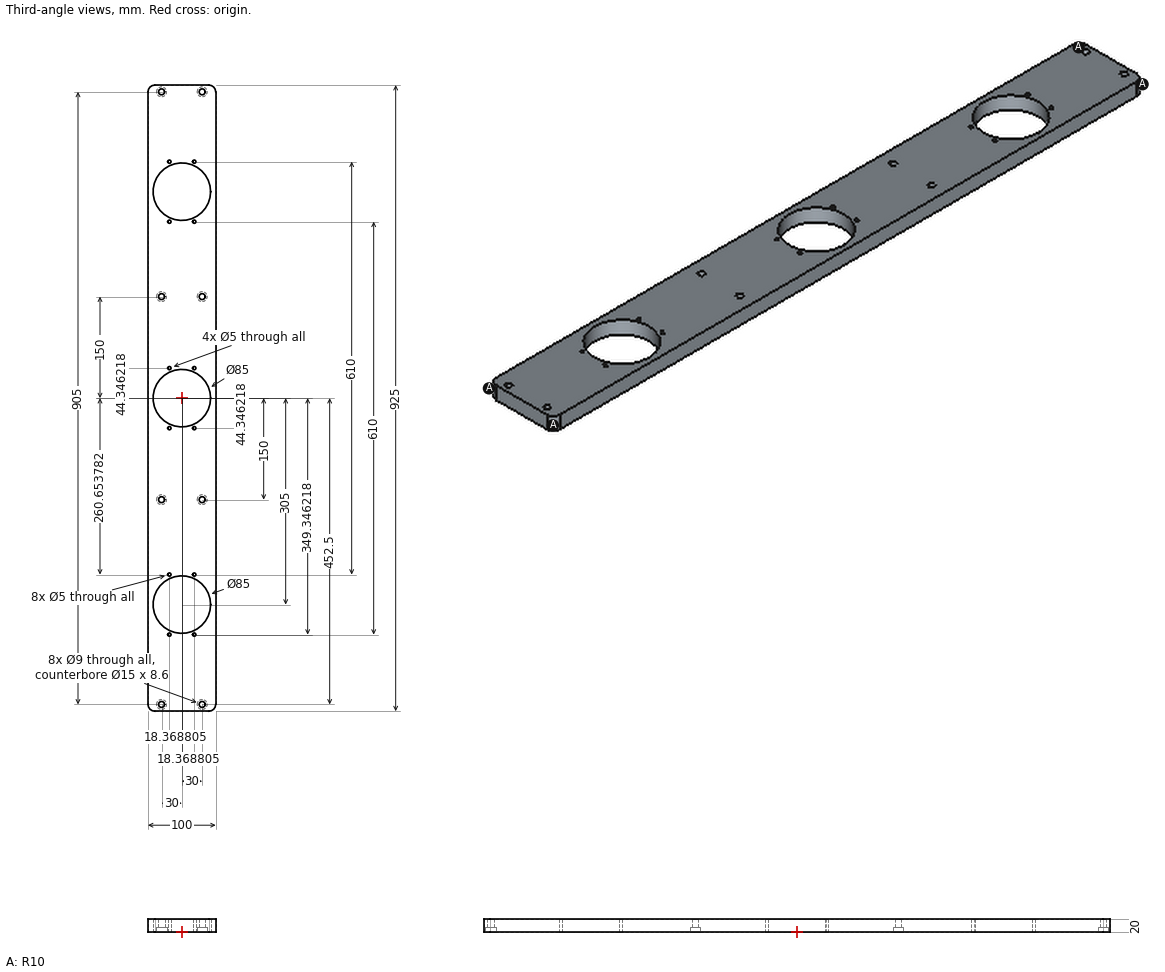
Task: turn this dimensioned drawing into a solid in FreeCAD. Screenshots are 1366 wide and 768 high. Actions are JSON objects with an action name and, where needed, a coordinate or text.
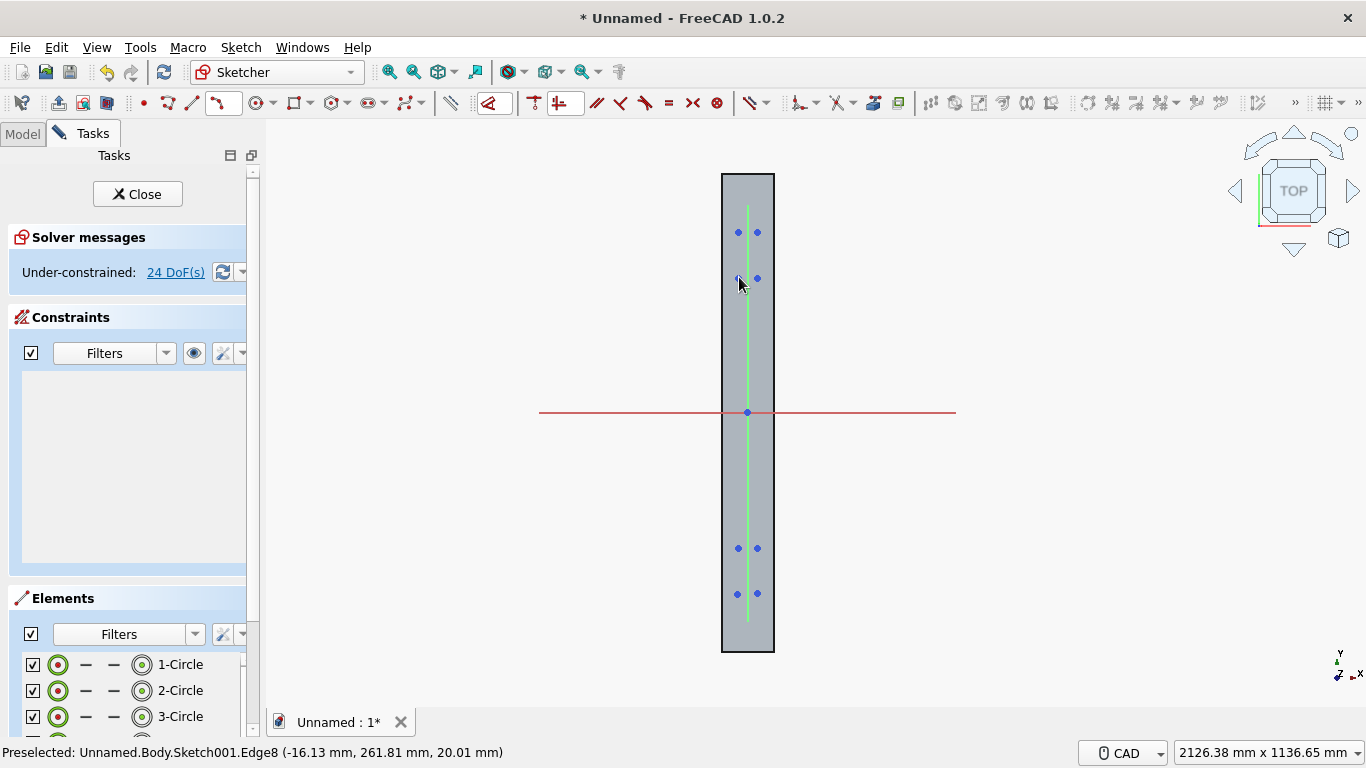
{"action": "scroll", "coordinate": [739, 547], "scroll_direction": "up", "scroll_amount": 11}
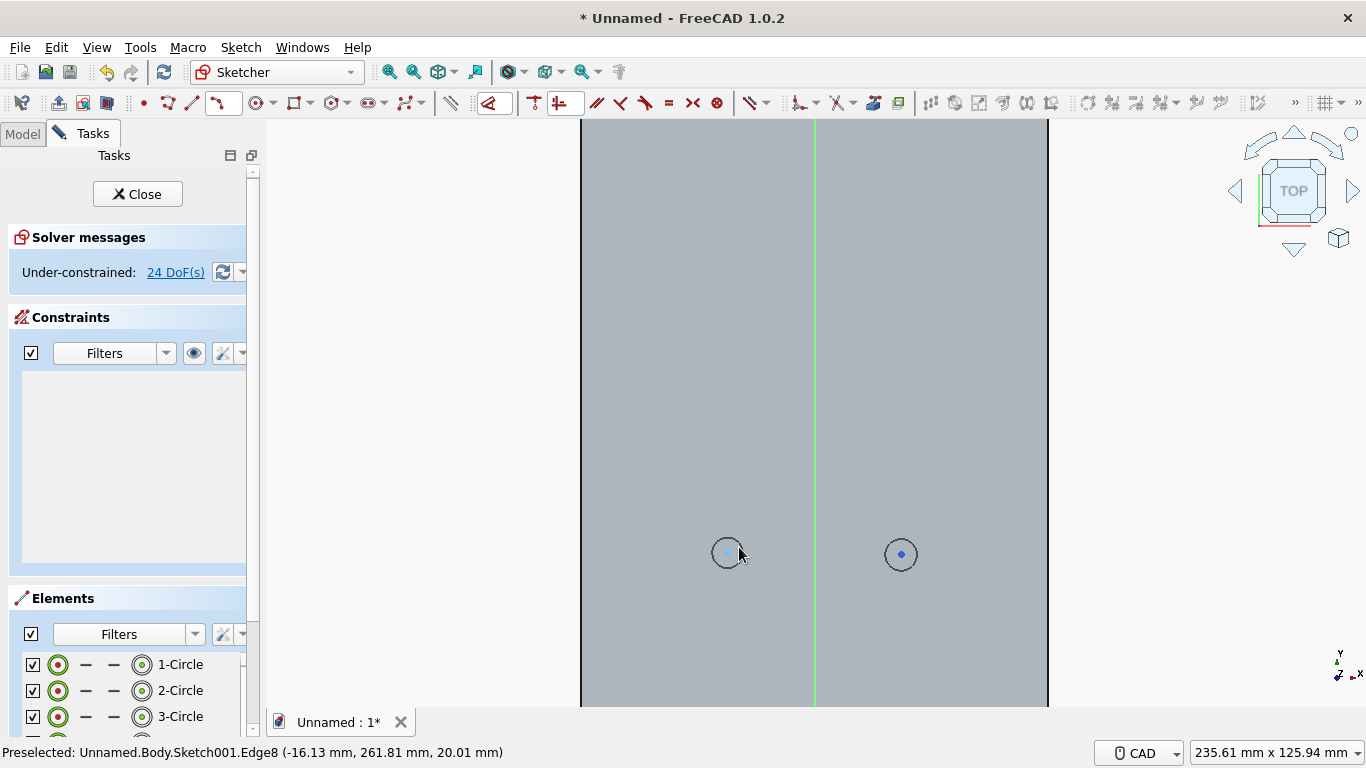
{"action": "left_click", "coordinate": [738, 542]}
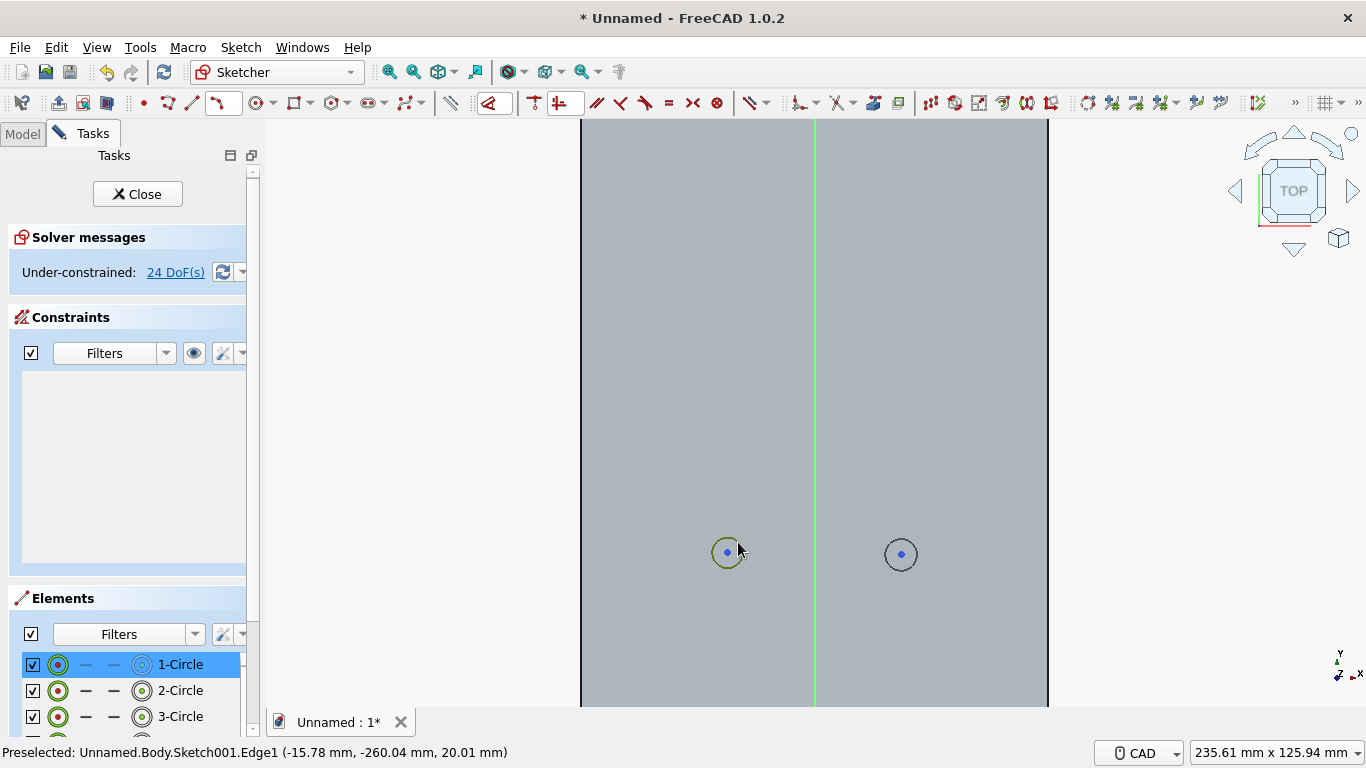
{"action": "left_click", "coordinate": [912, 544]}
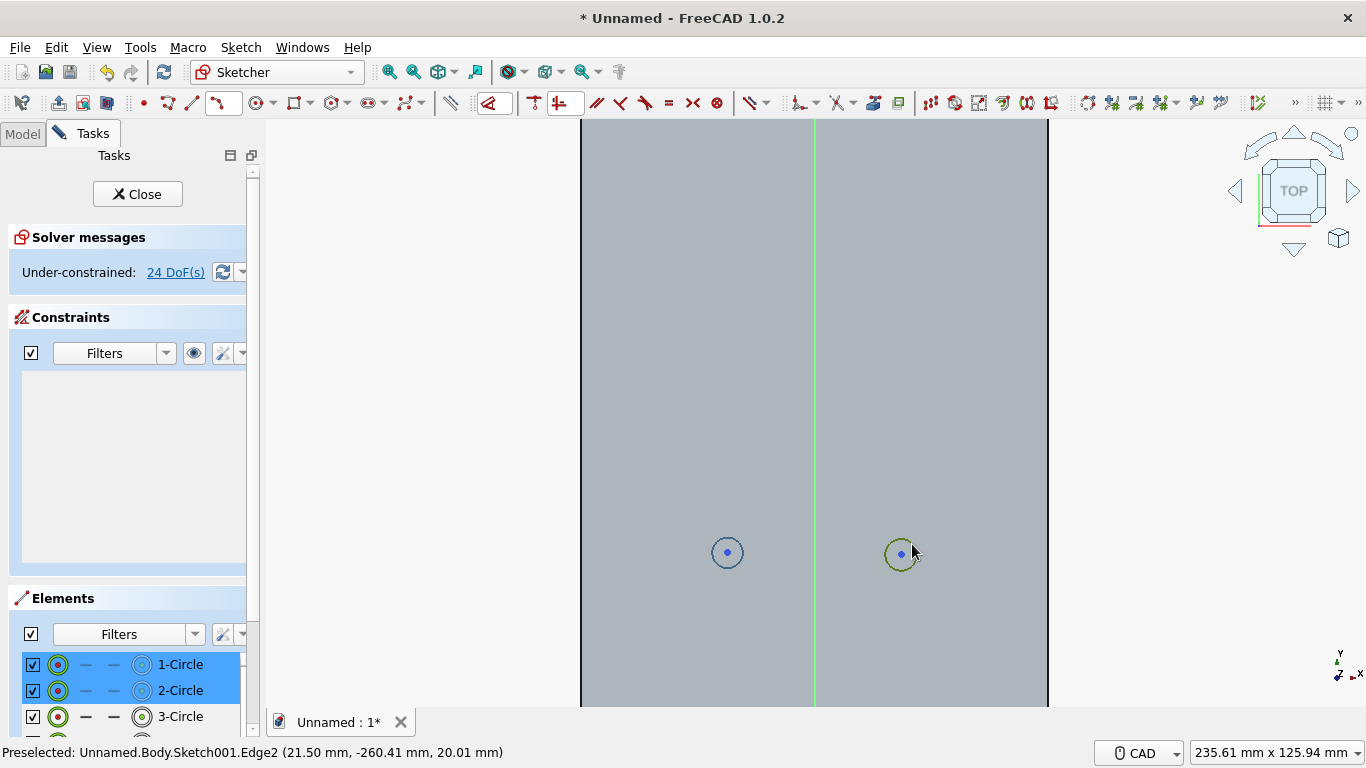
{"action": "scroll", "coordinate": [739, 548], "scroll_direction": "down", "scroll_amount": 11}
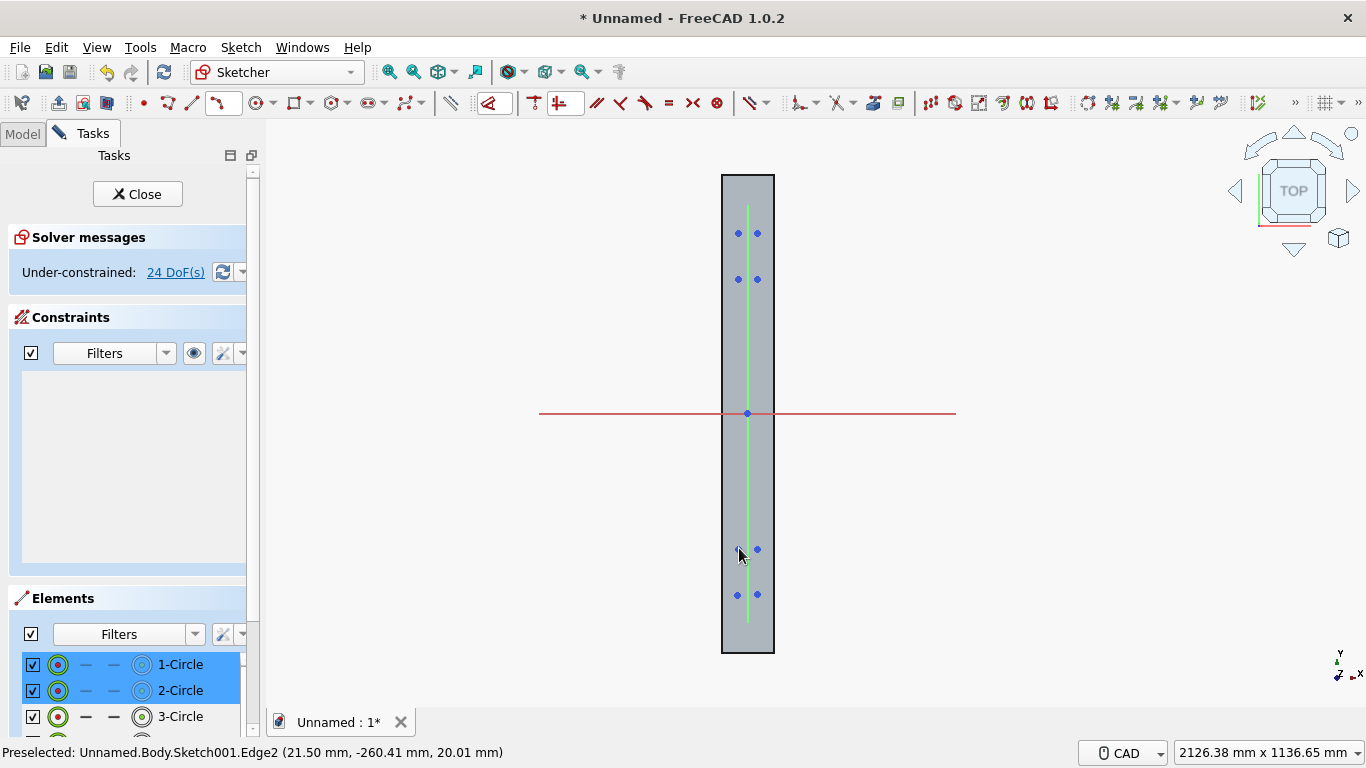
{"action": "scroll", "coordinate": [758, 594], "scroll_direction": "up", "scroll_amount": 12}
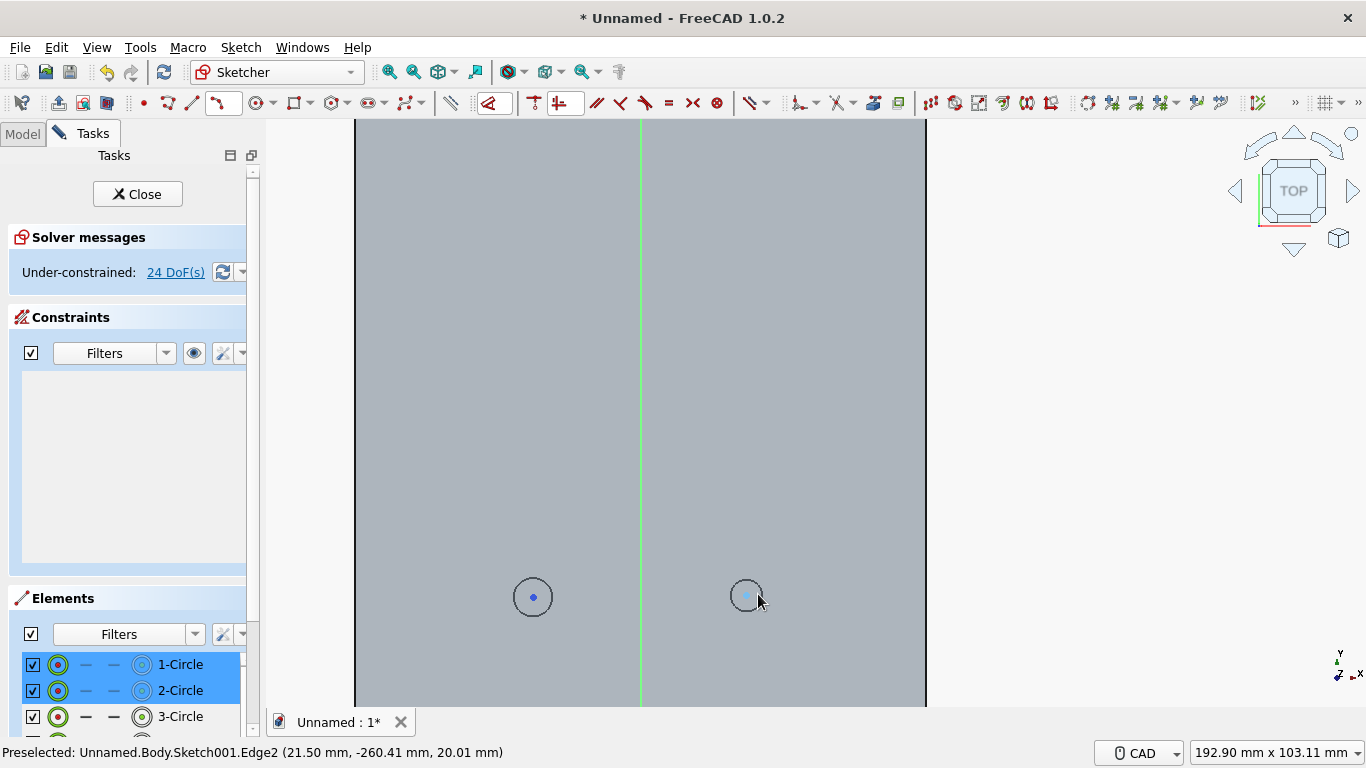
{"action": "left_click", "coordinate": [758, 584]}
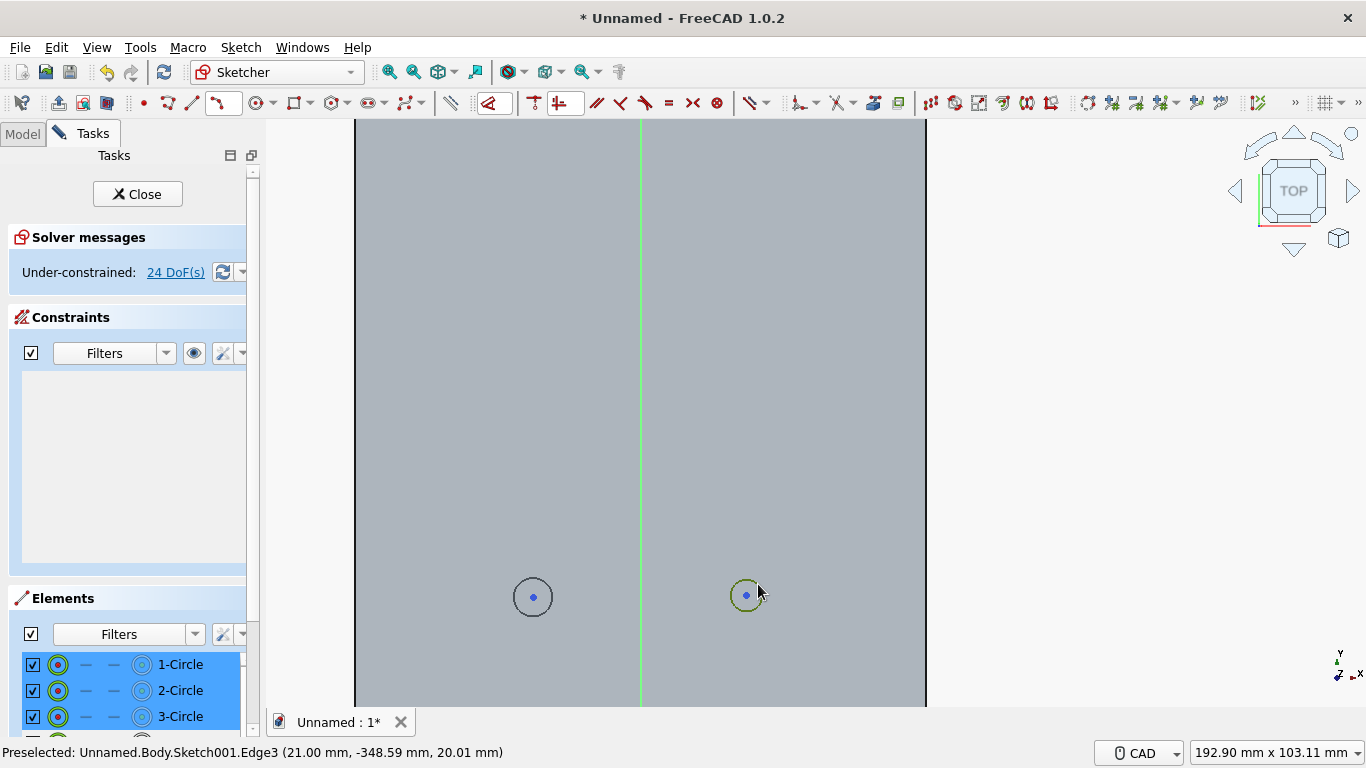
{"action": "left_click", "coordinate": [547, 584]}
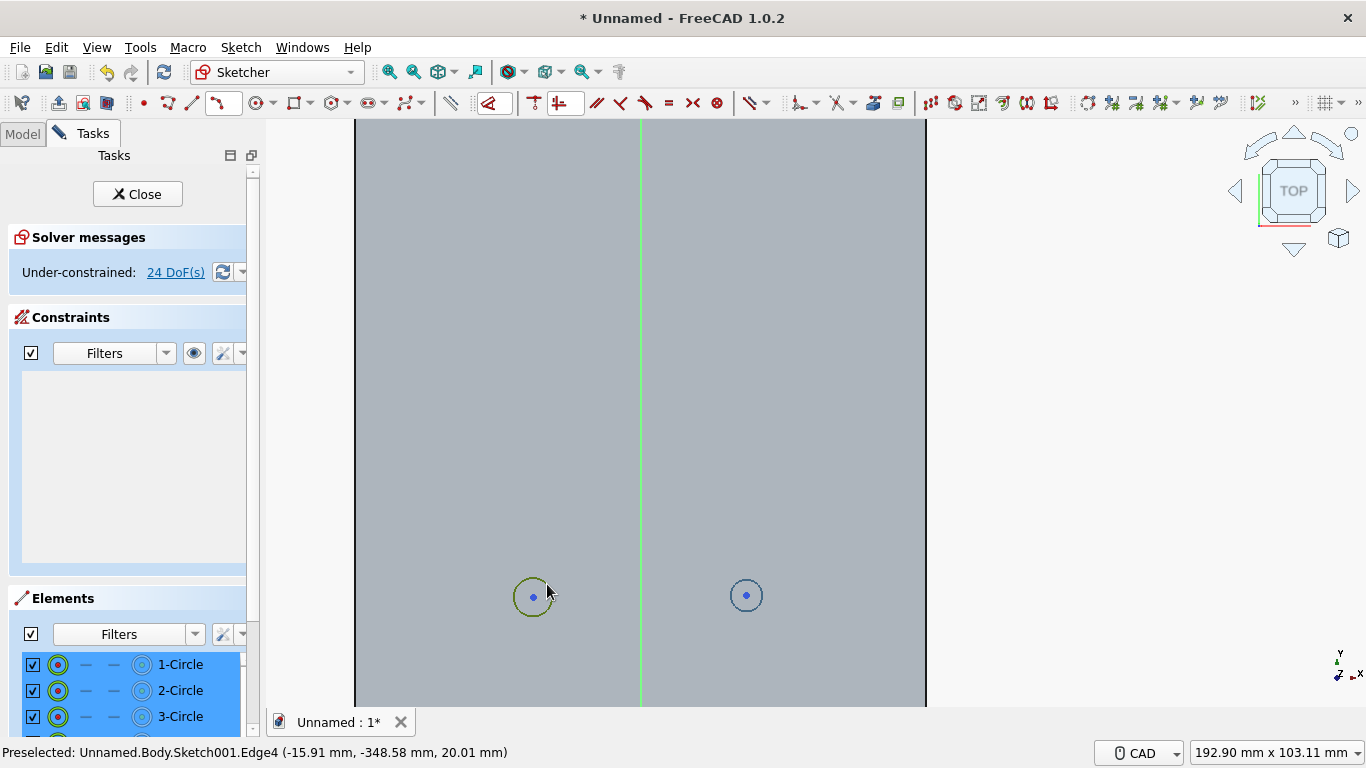
{"action": "scroll", "coordinate": [758, 594], "scroll_direction": "down", "scroll_amount": 12}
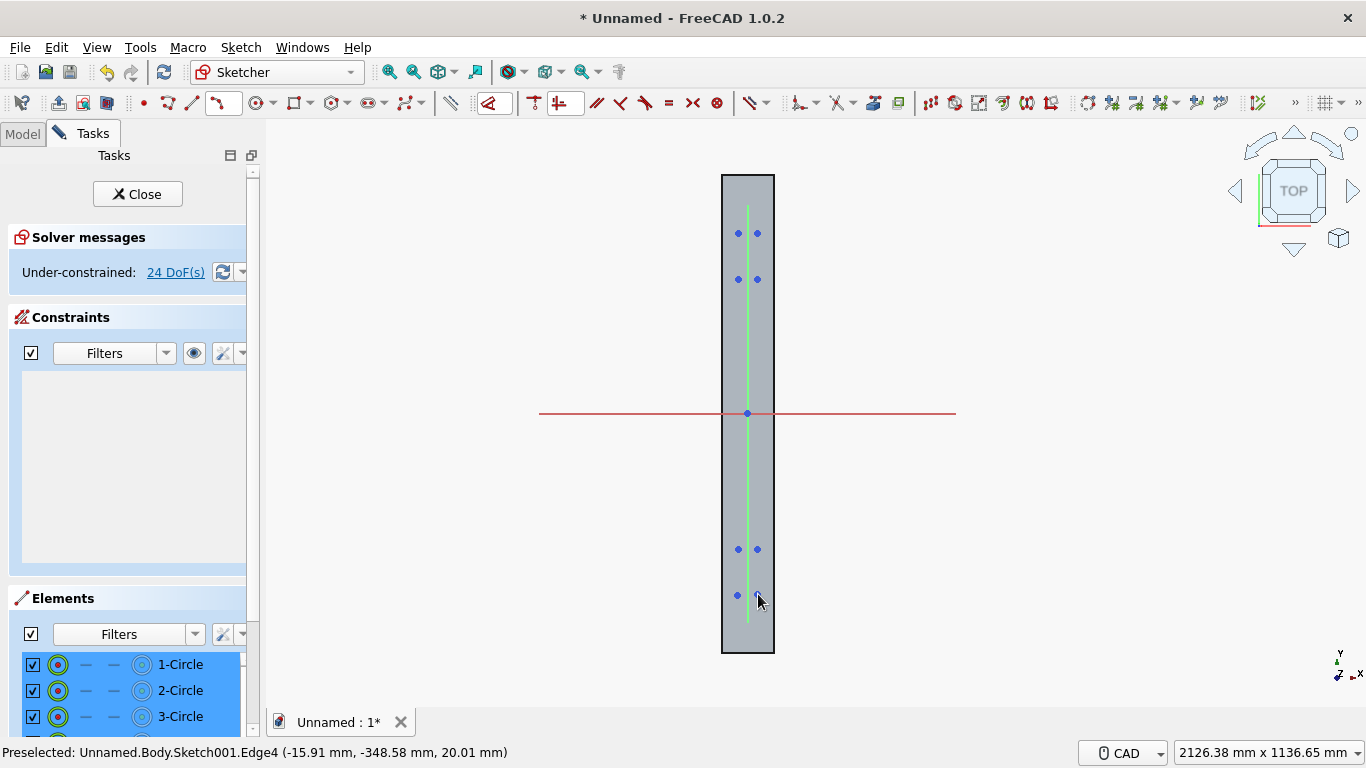
{"action": "scroll", "coordinate": [758, 232], "scroll_direction": "up", "scroll_amount": 11}